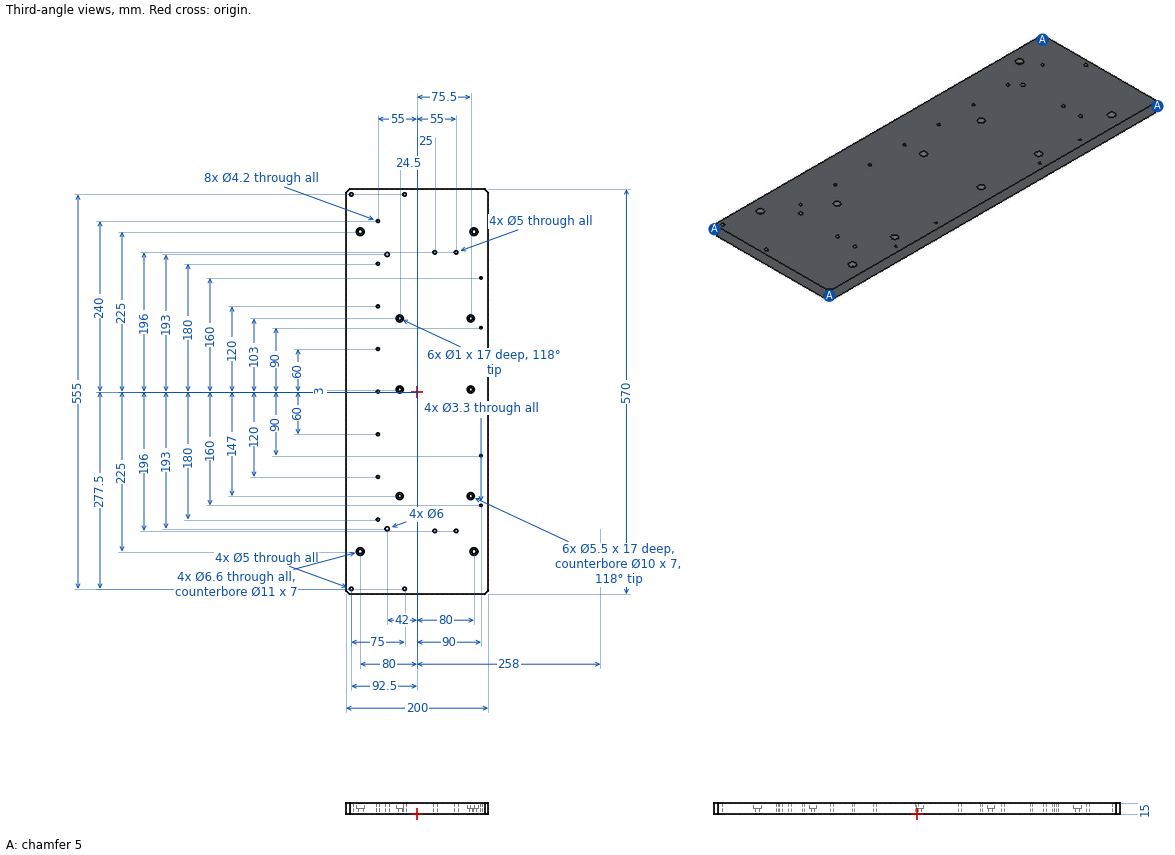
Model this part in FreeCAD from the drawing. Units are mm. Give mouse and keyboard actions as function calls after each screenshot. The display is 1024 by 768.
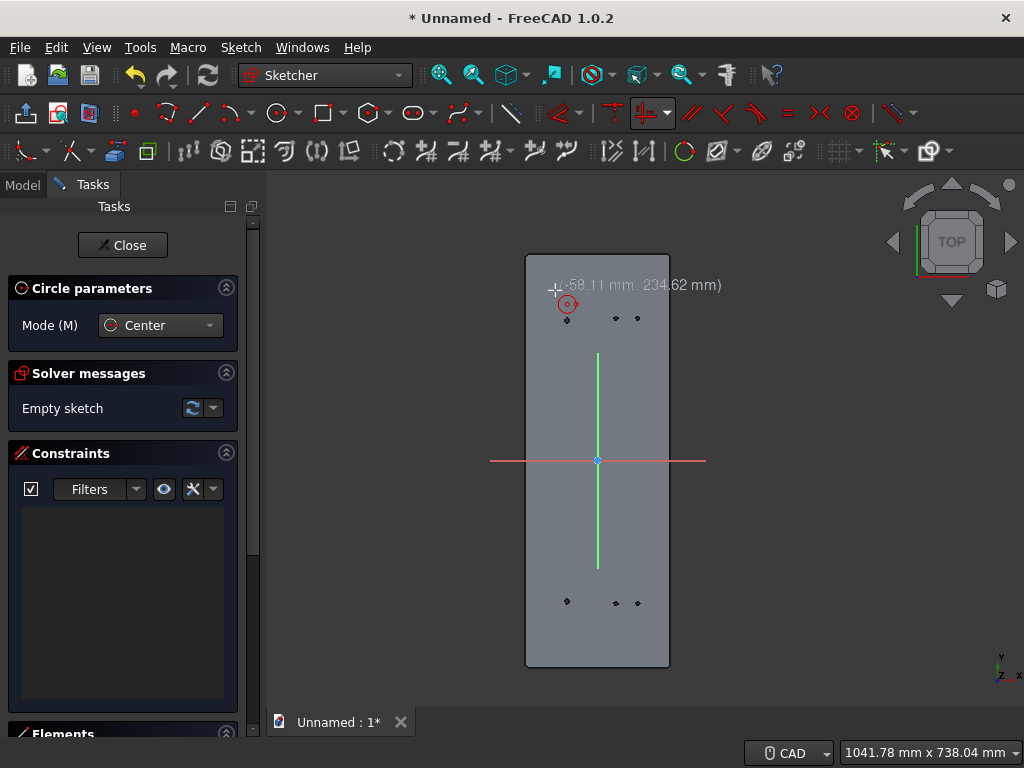
click(558, 286)
move(559, 285)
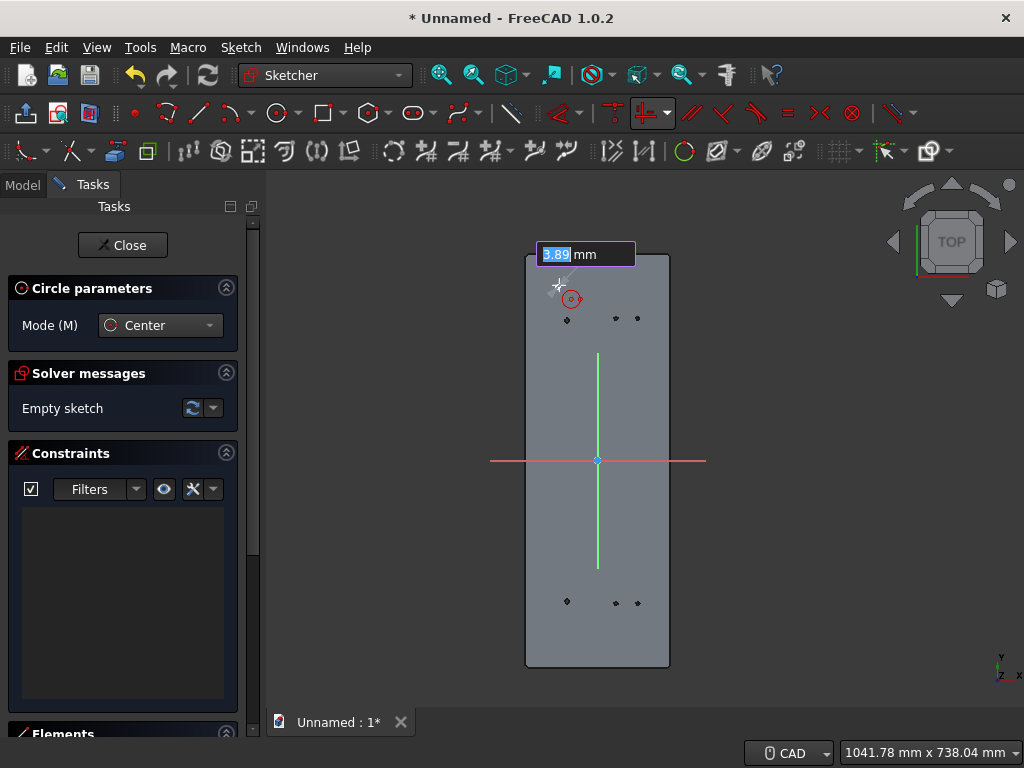
text(4.2)
key(Return)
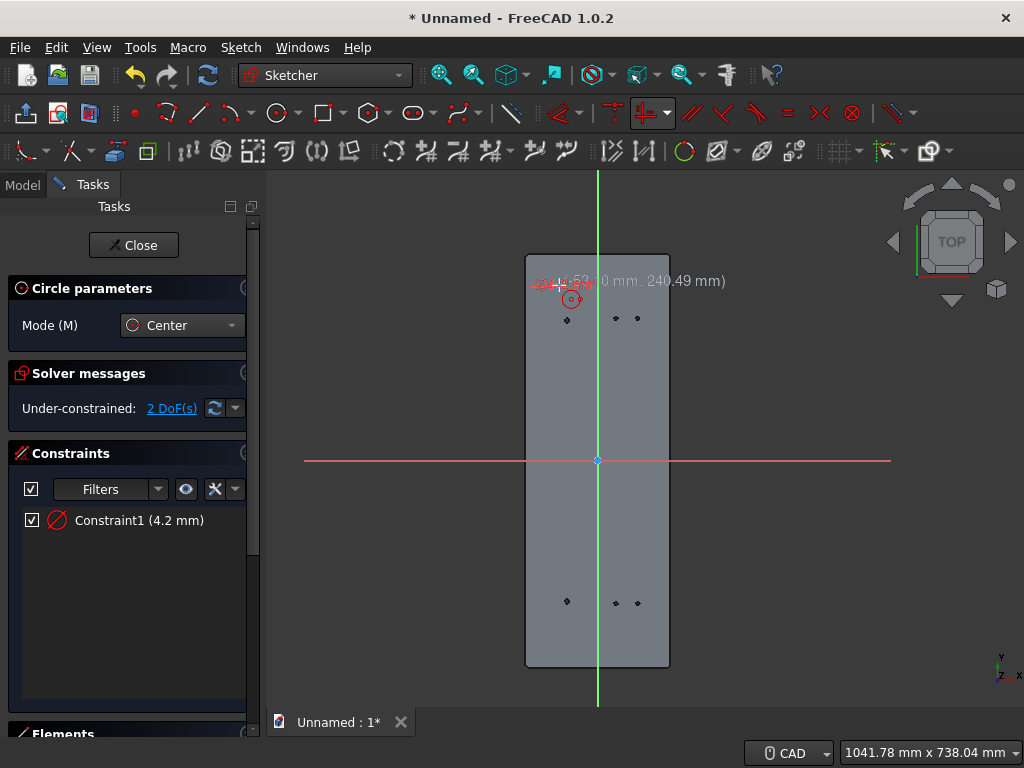
scroll(558, 330, up, 14)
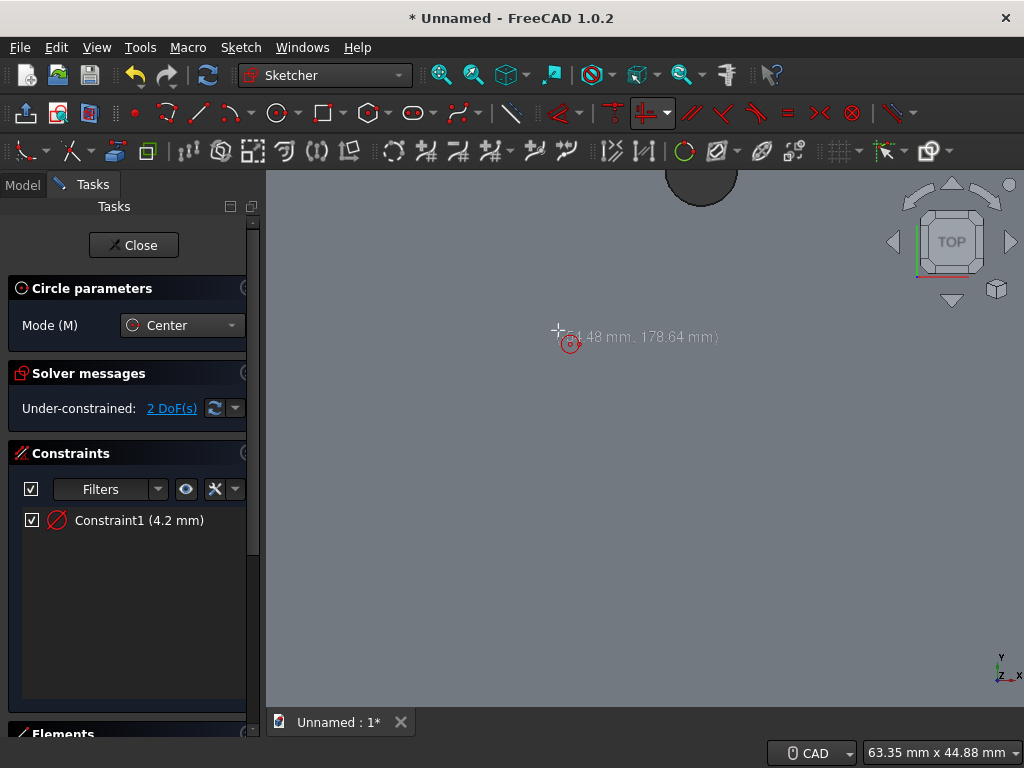
scroll(558, 330, down, 14)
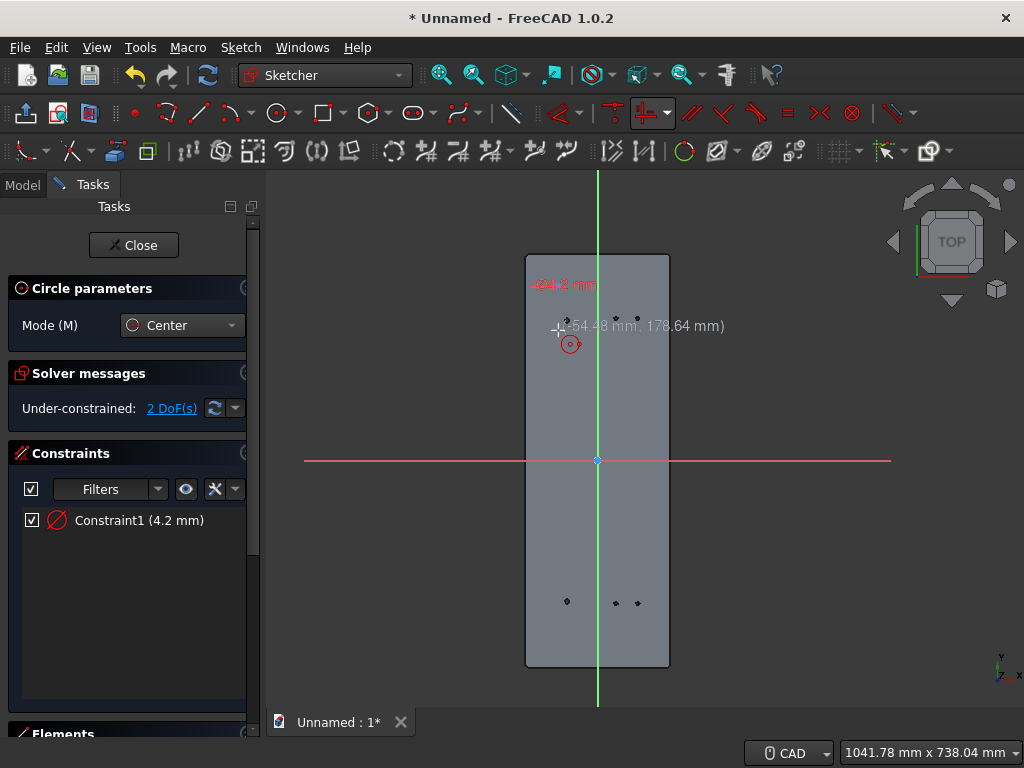
click(558, 330)
move(559, 329)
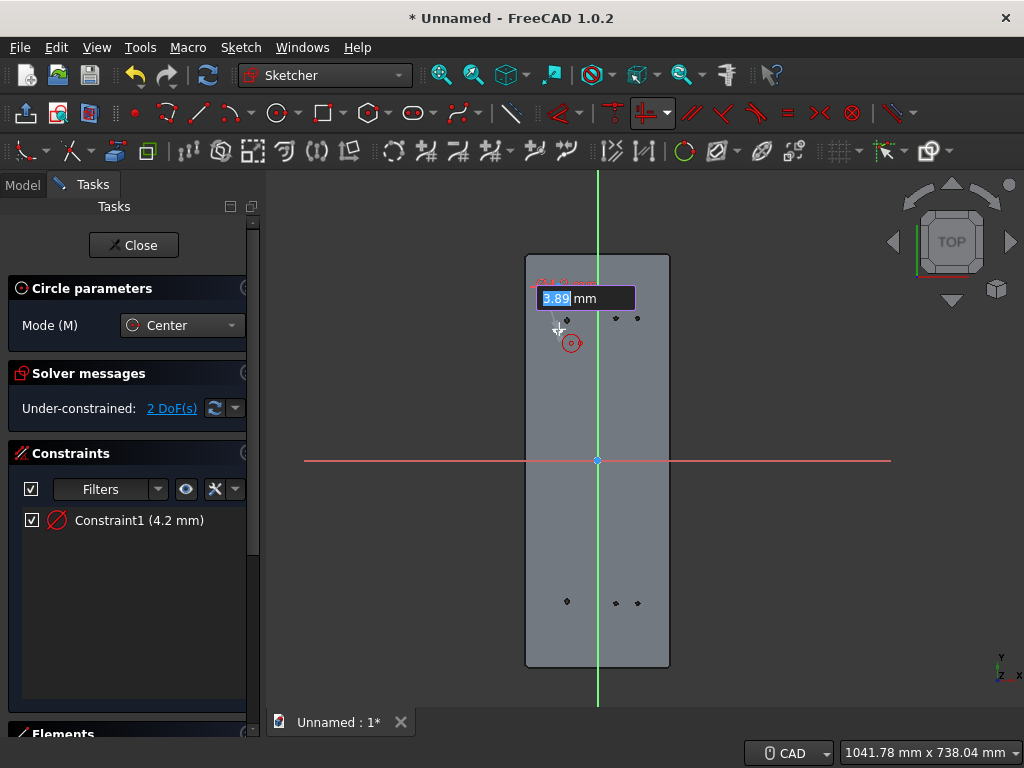
text(4.2)
key(Return)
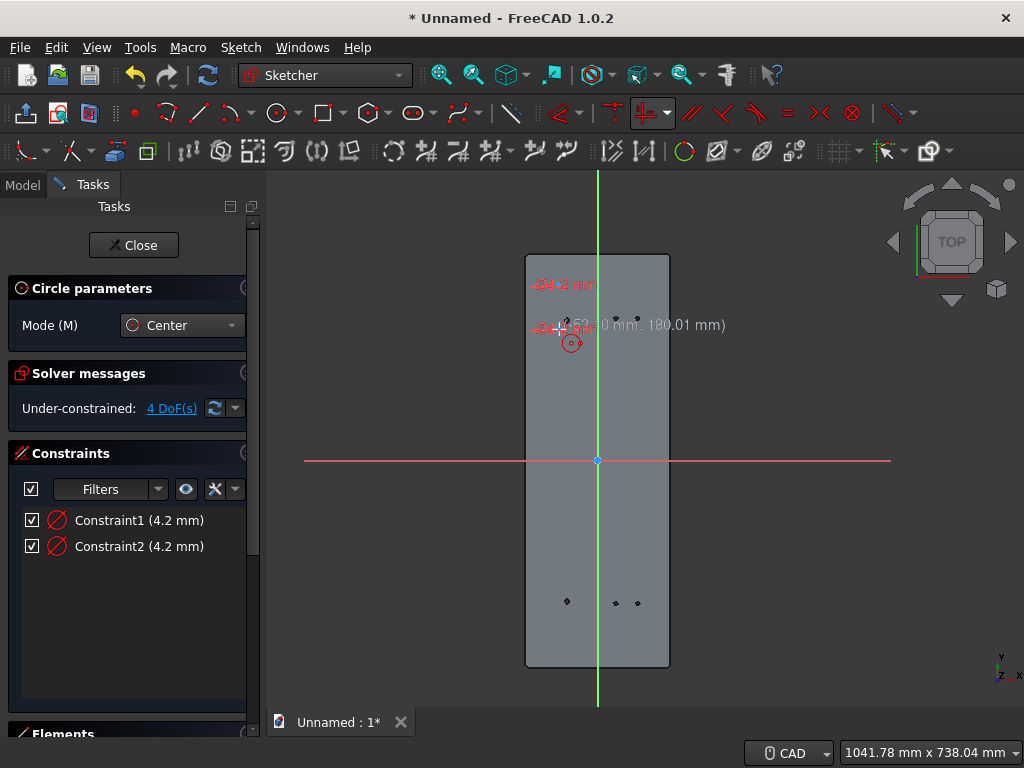
scroll(558, 374, up, 14)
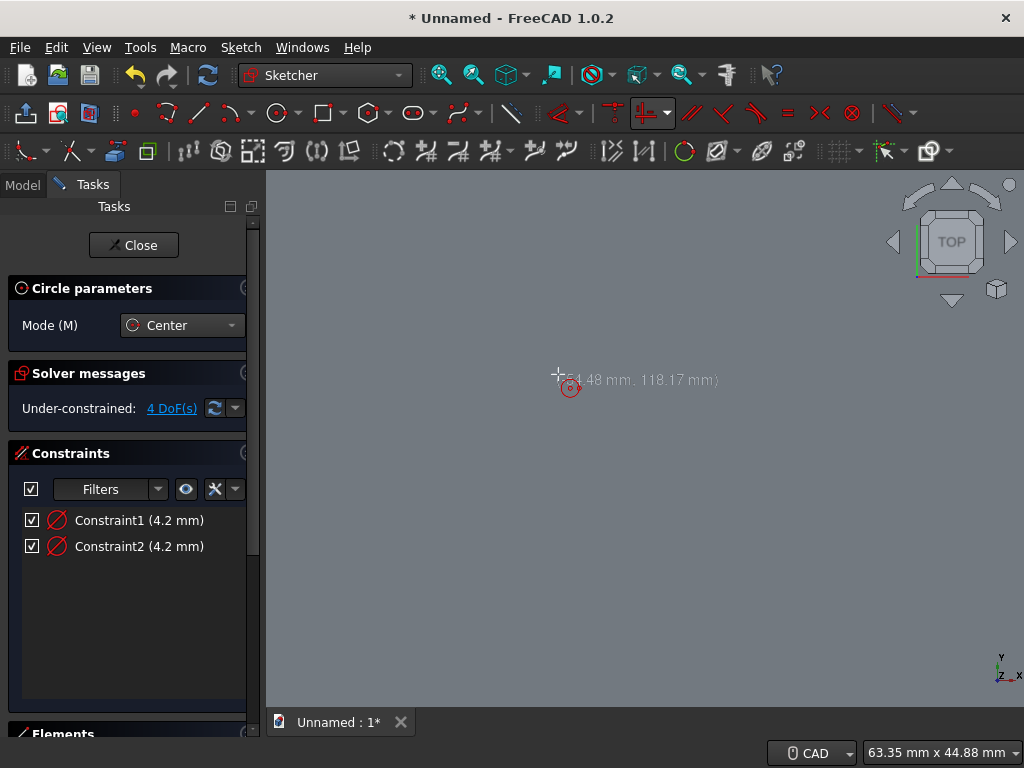
scroll(558, 374, down, 14)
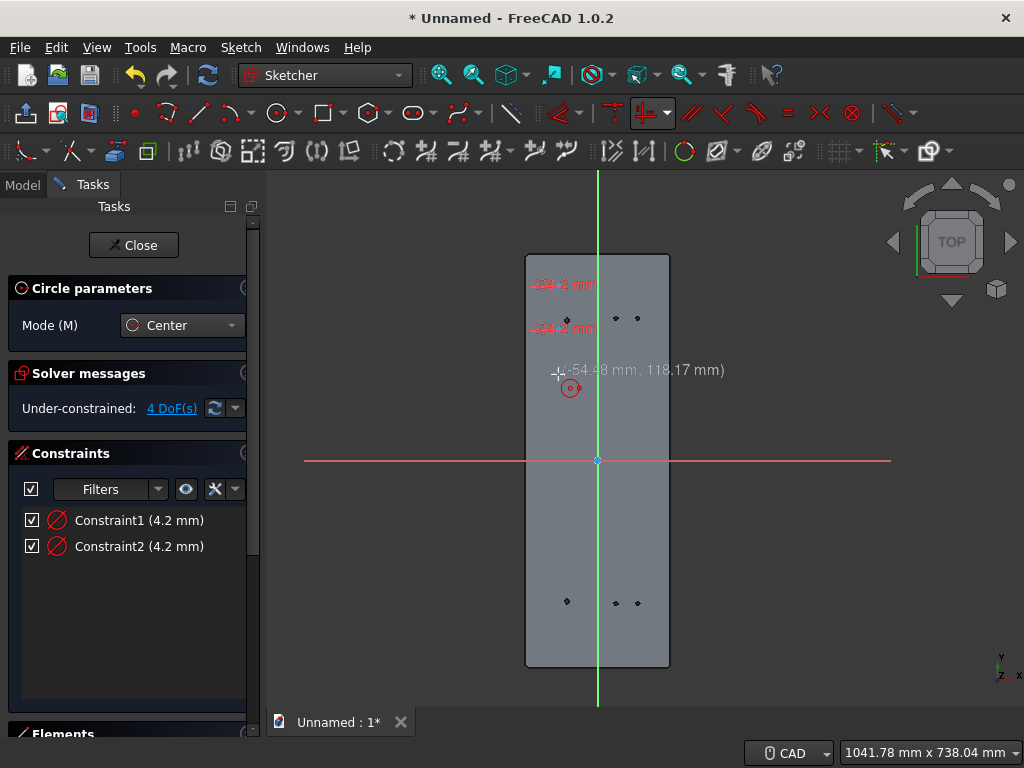
click(558, 374)
move(559, 373)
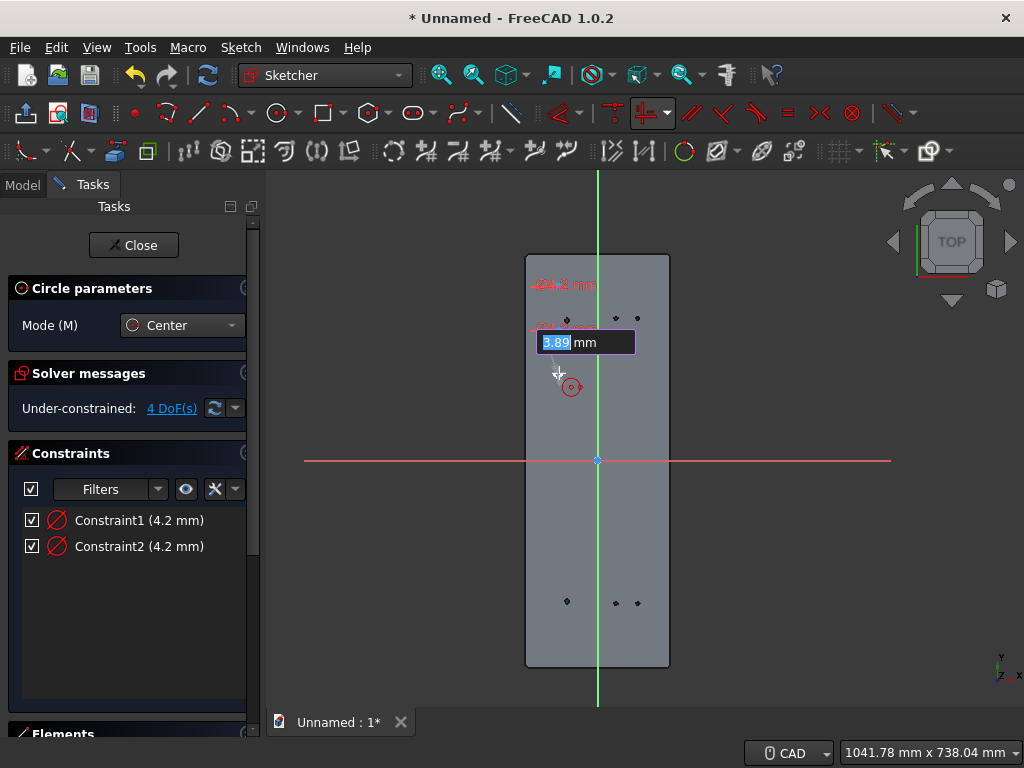
text(4.2)
key(Return)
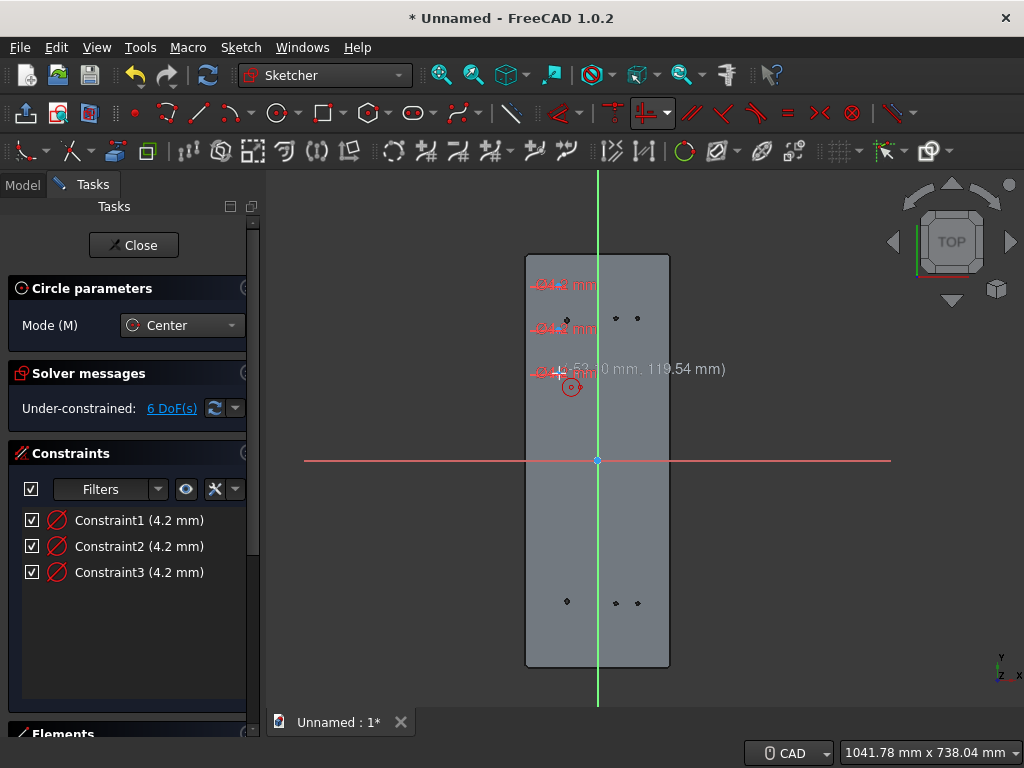
scroll(558, 417, up, 14)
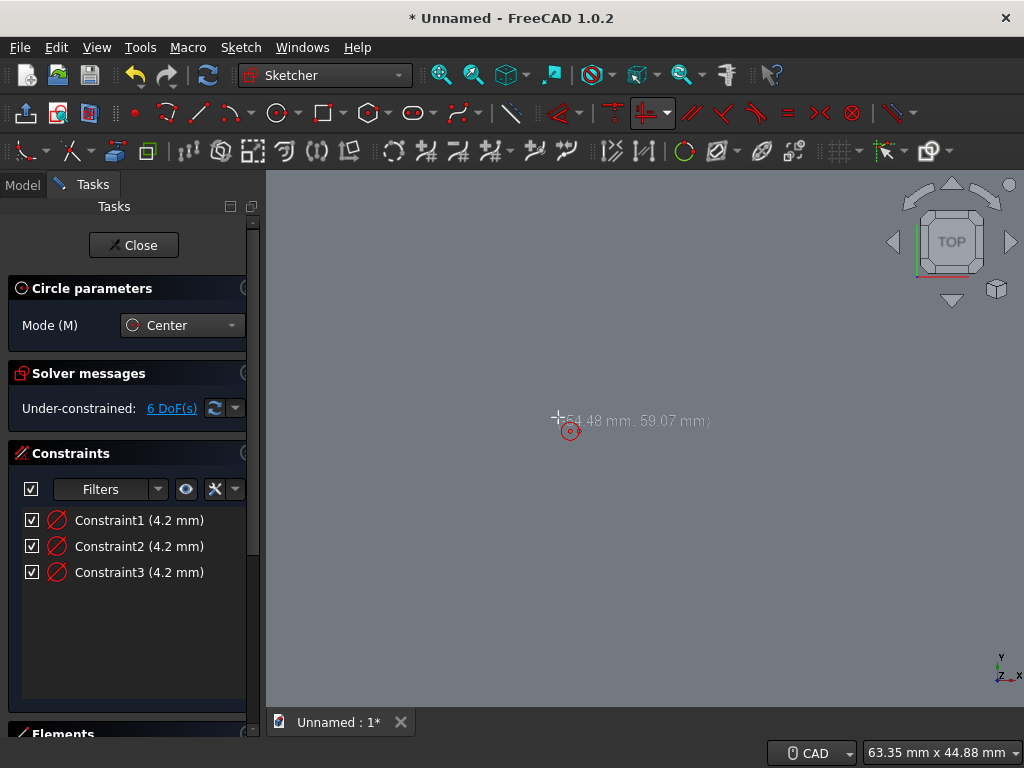
scroll(558, 417, down, 14)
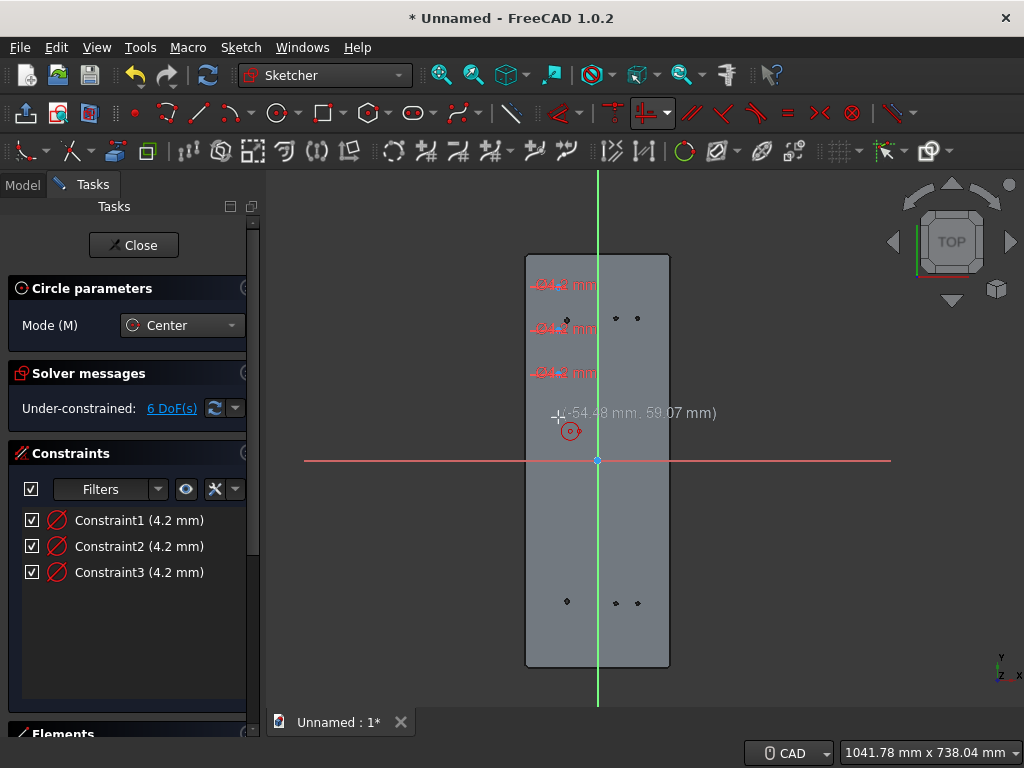
click(558, 417)
move(559, 416)